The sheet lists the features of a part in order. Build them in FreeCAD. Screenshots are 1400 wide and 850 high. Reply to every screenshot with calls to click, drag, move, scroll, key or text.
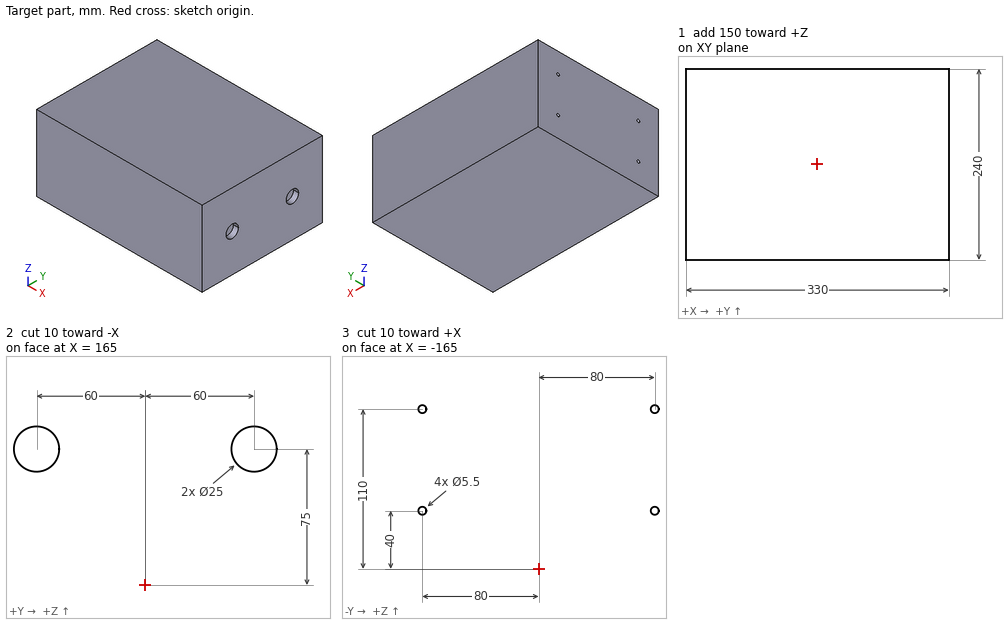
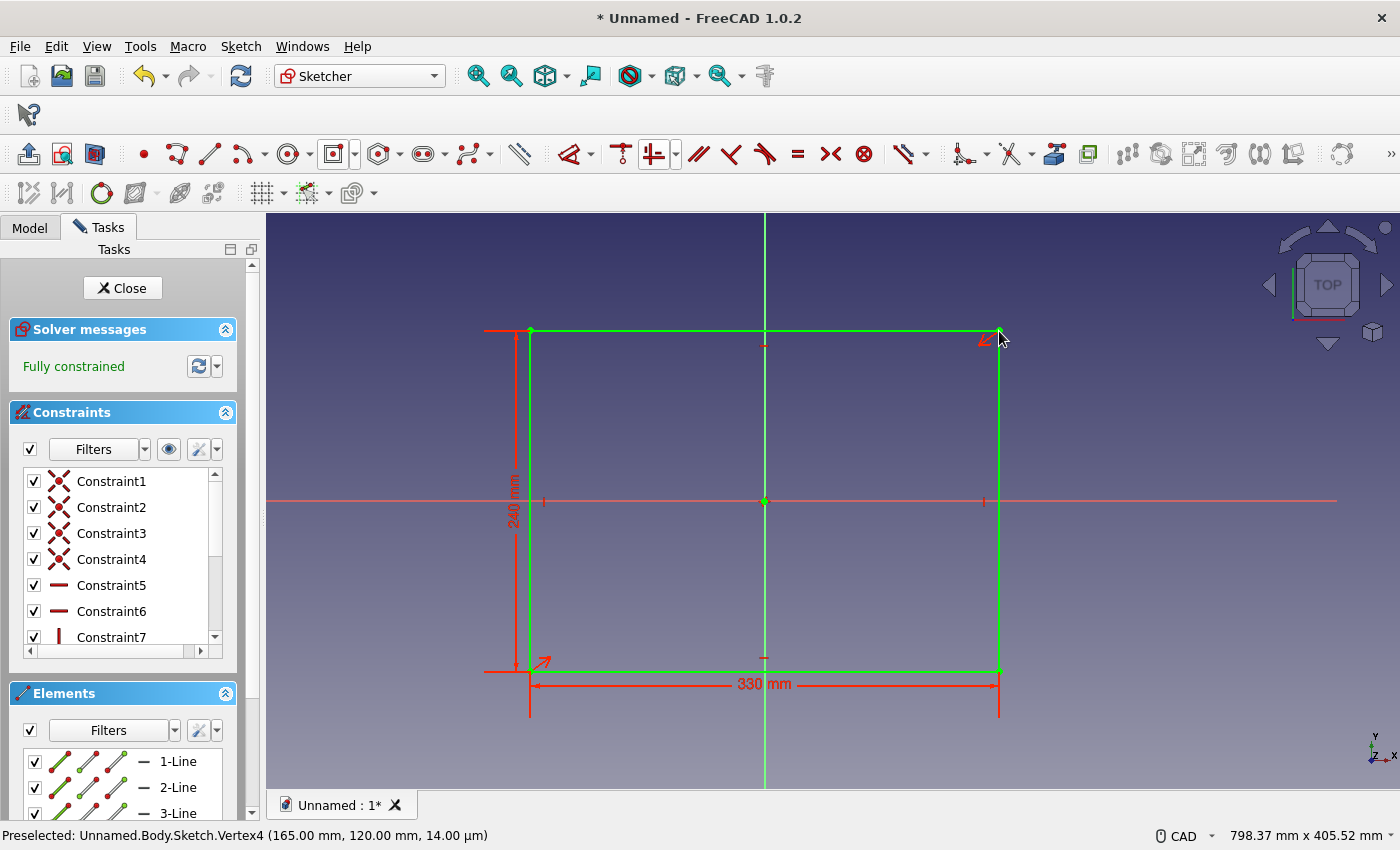
click(123, 288)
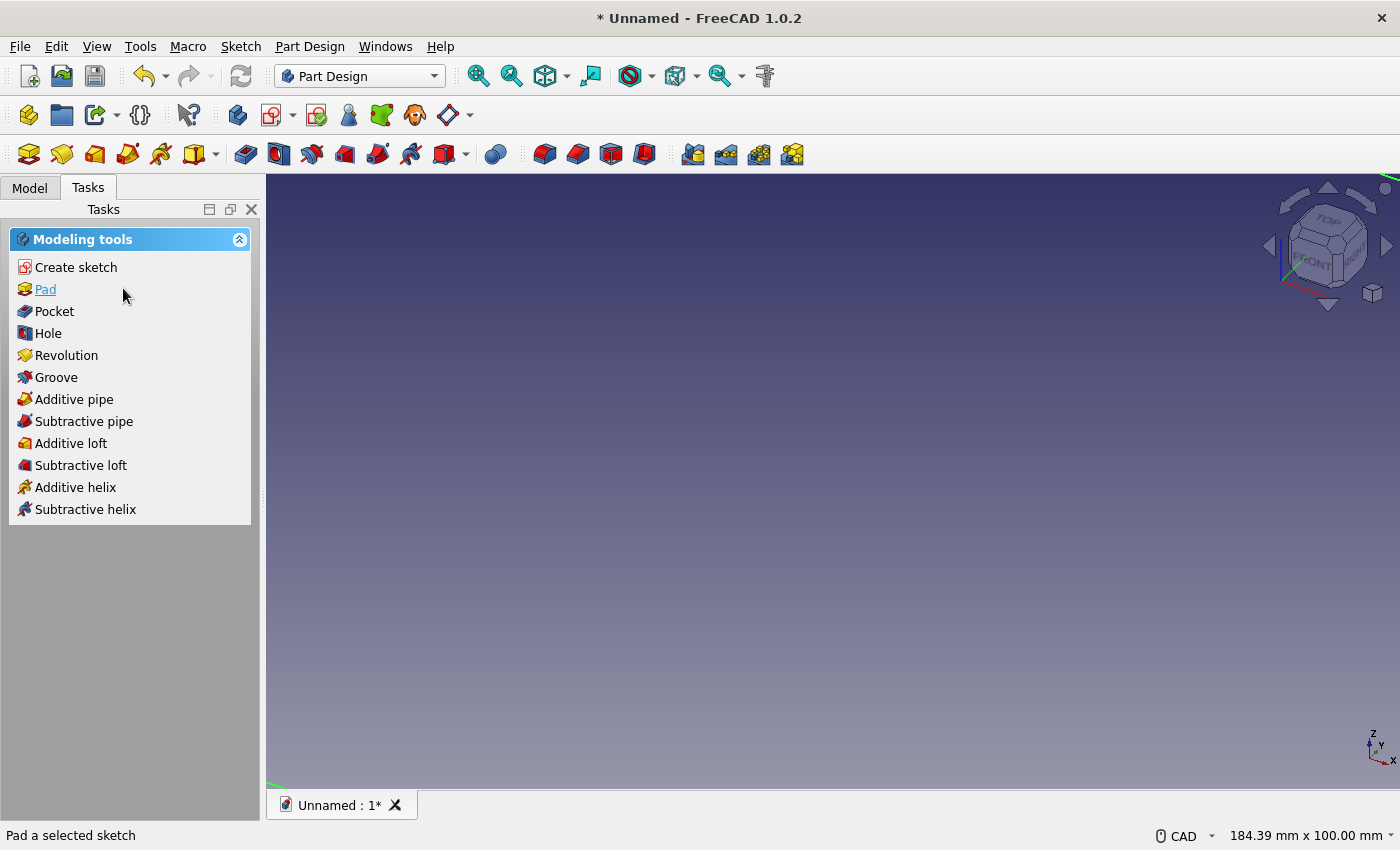
click(29, 154)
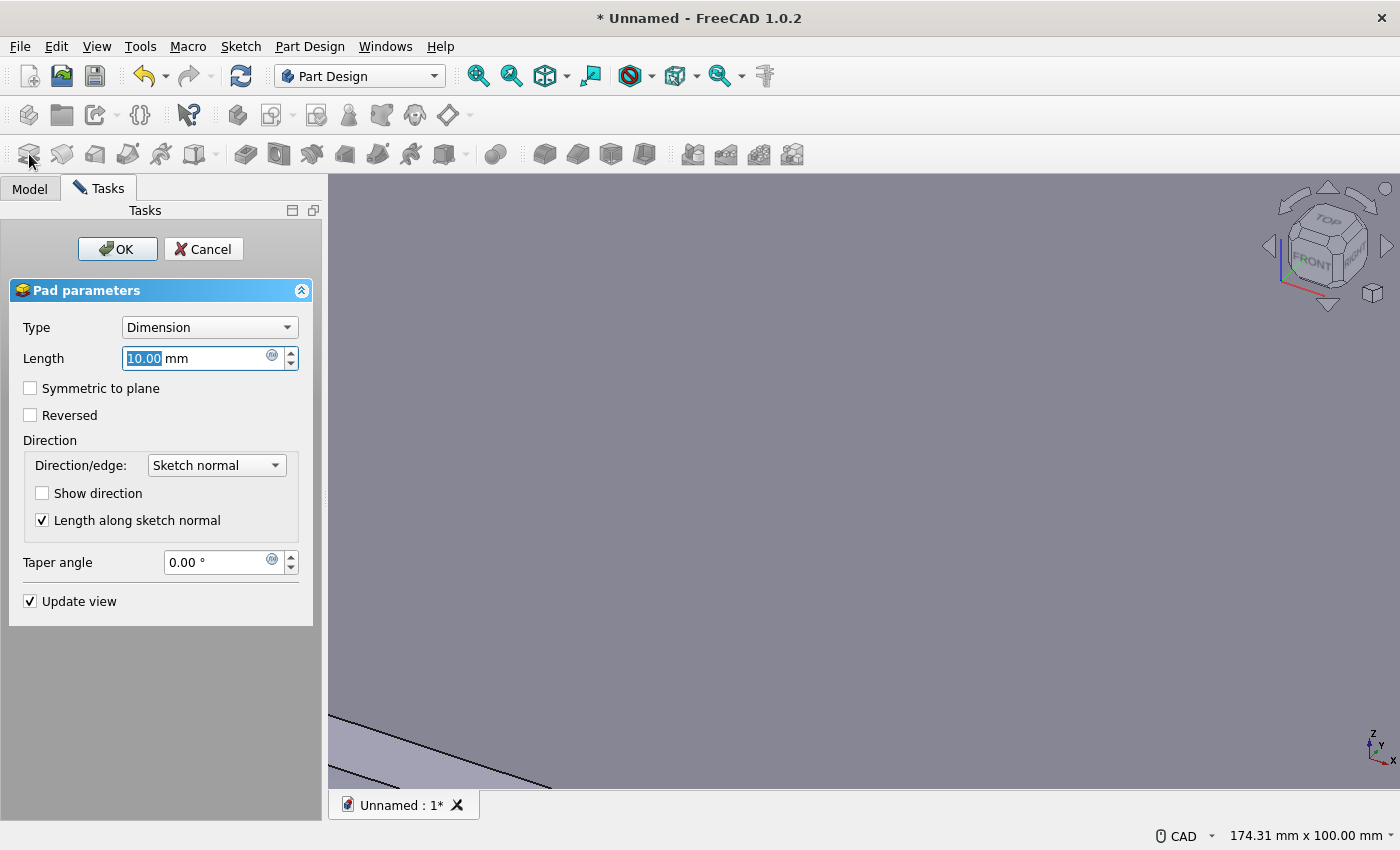
text(150)
key(Tab)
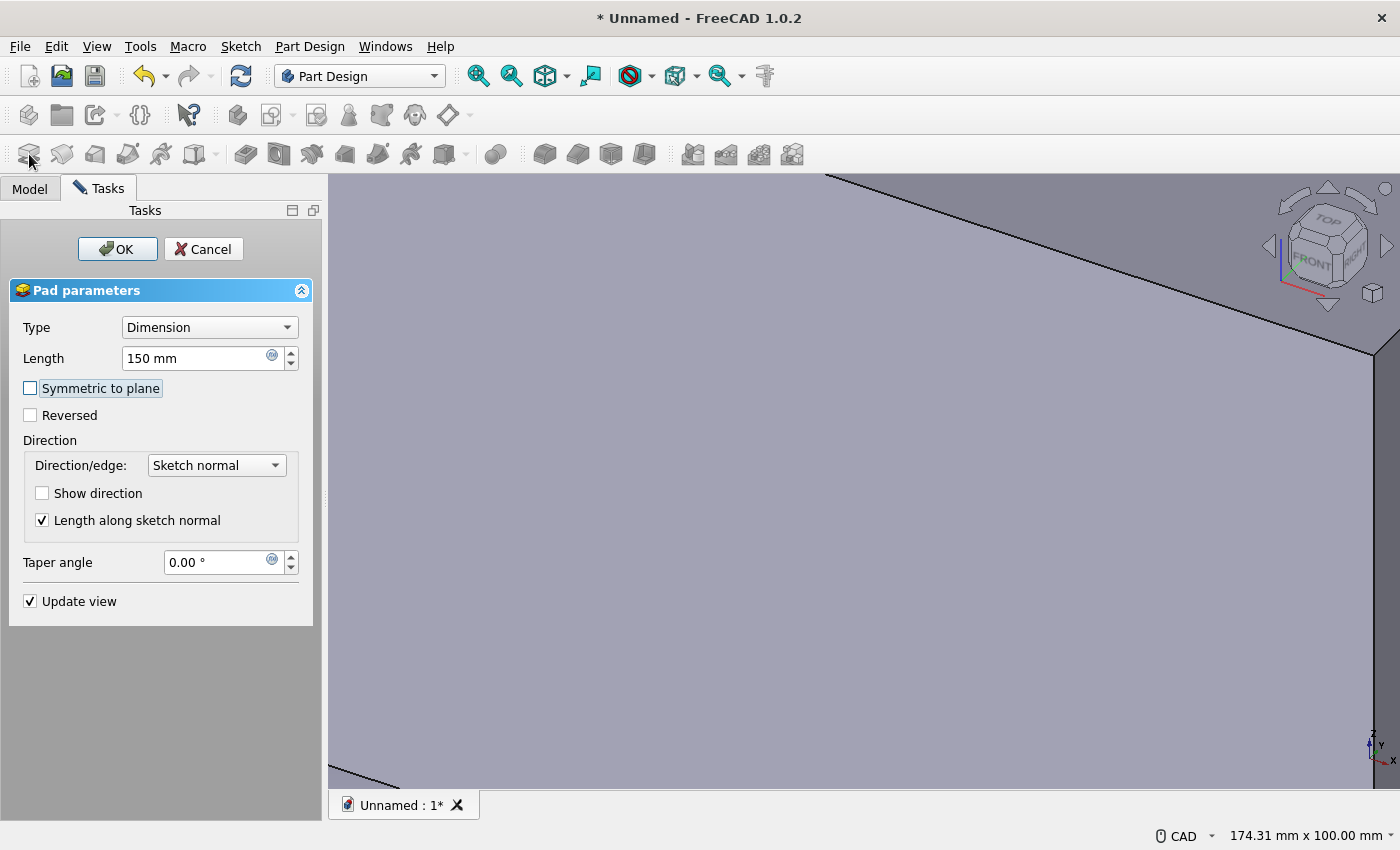
click(118, 249)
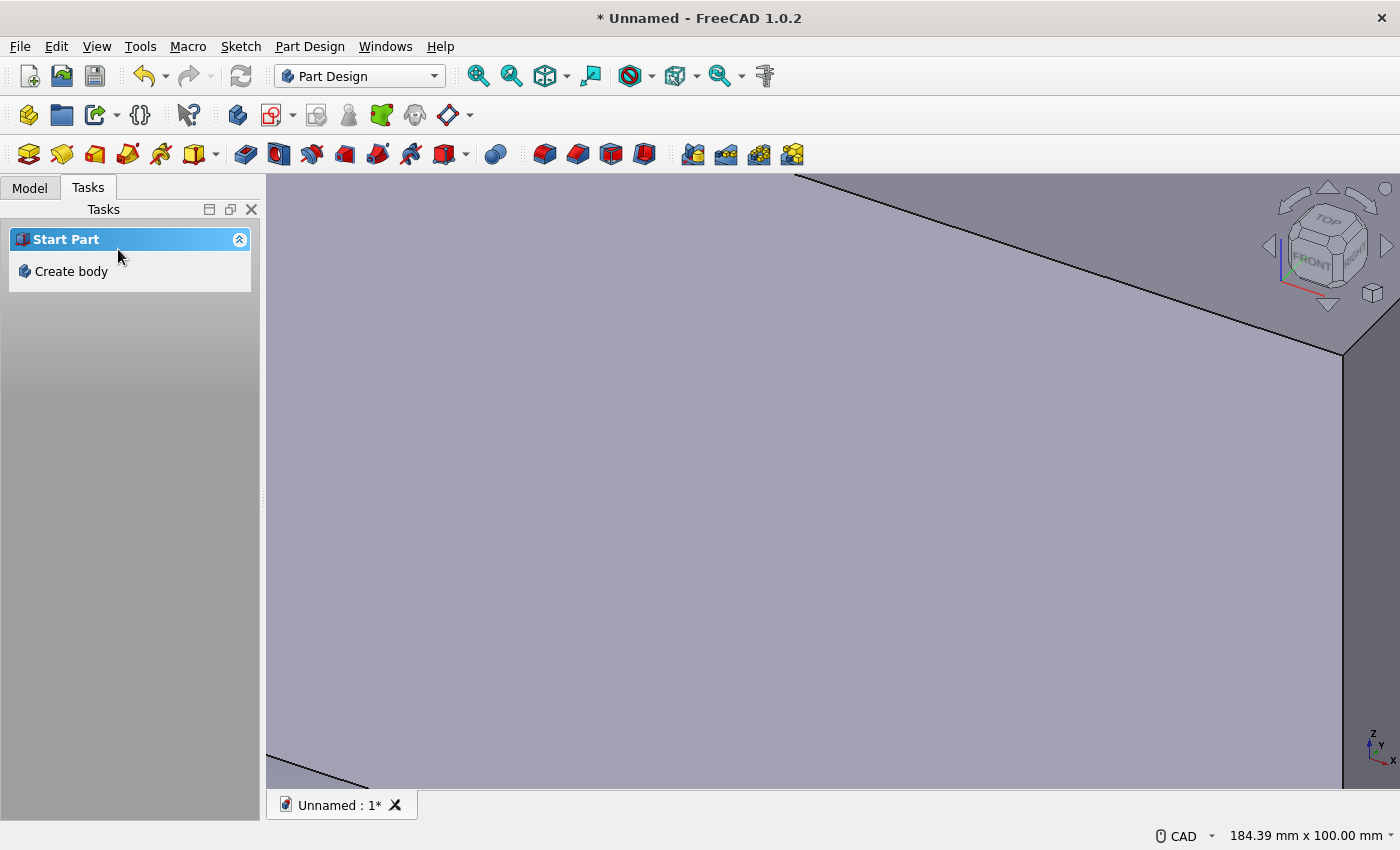
click(479, 76)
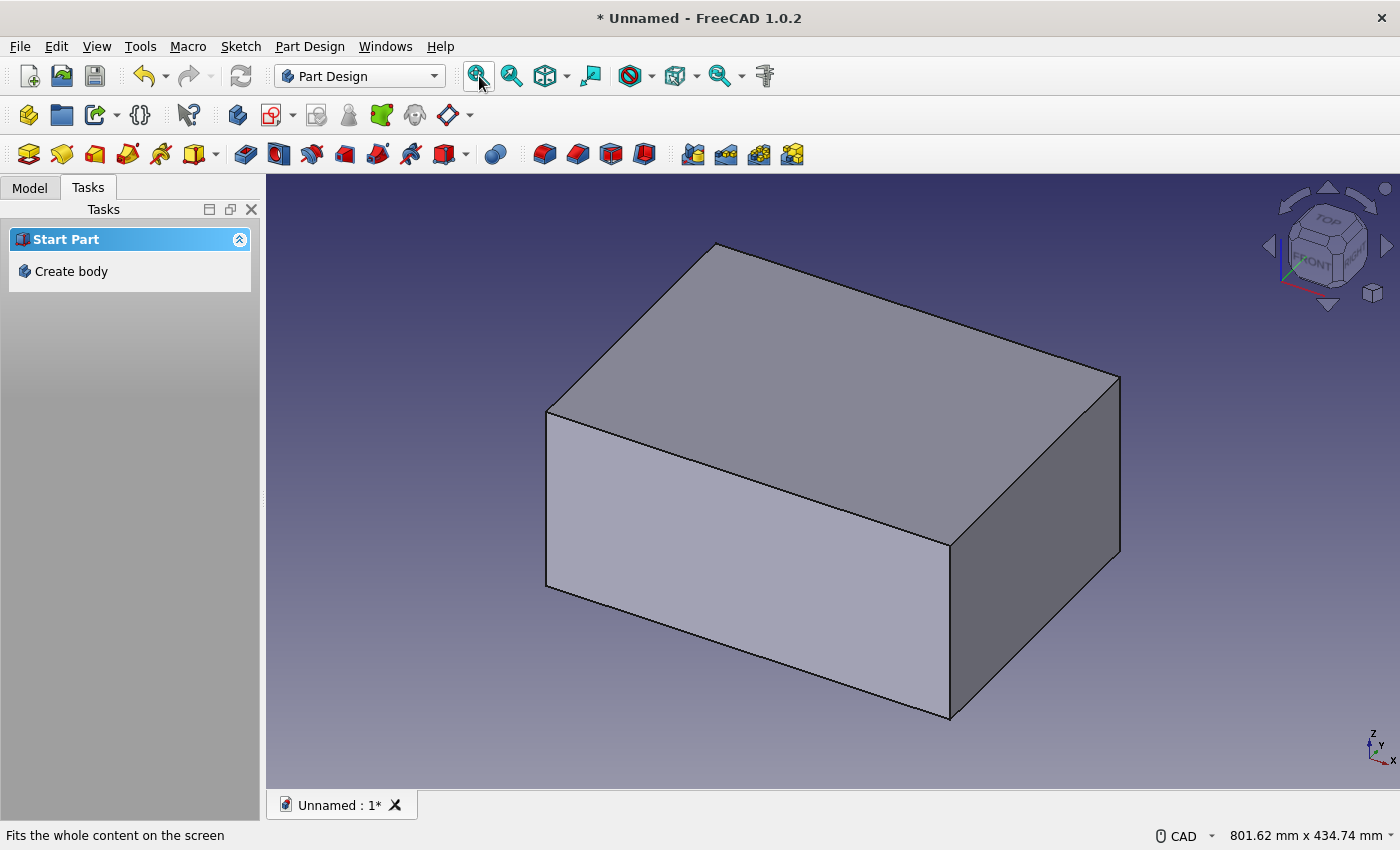
click(1059, 523)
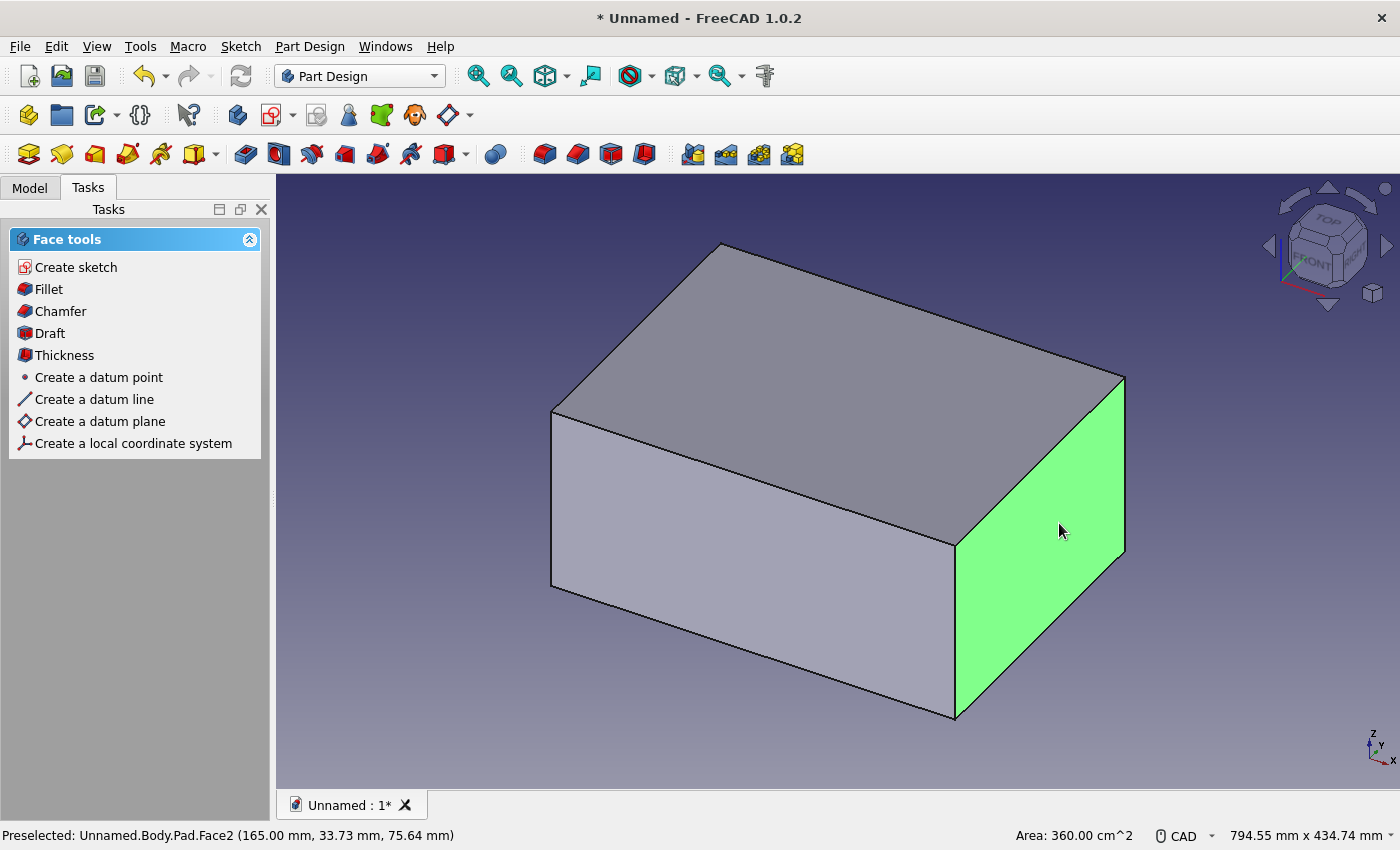
click(270, 116)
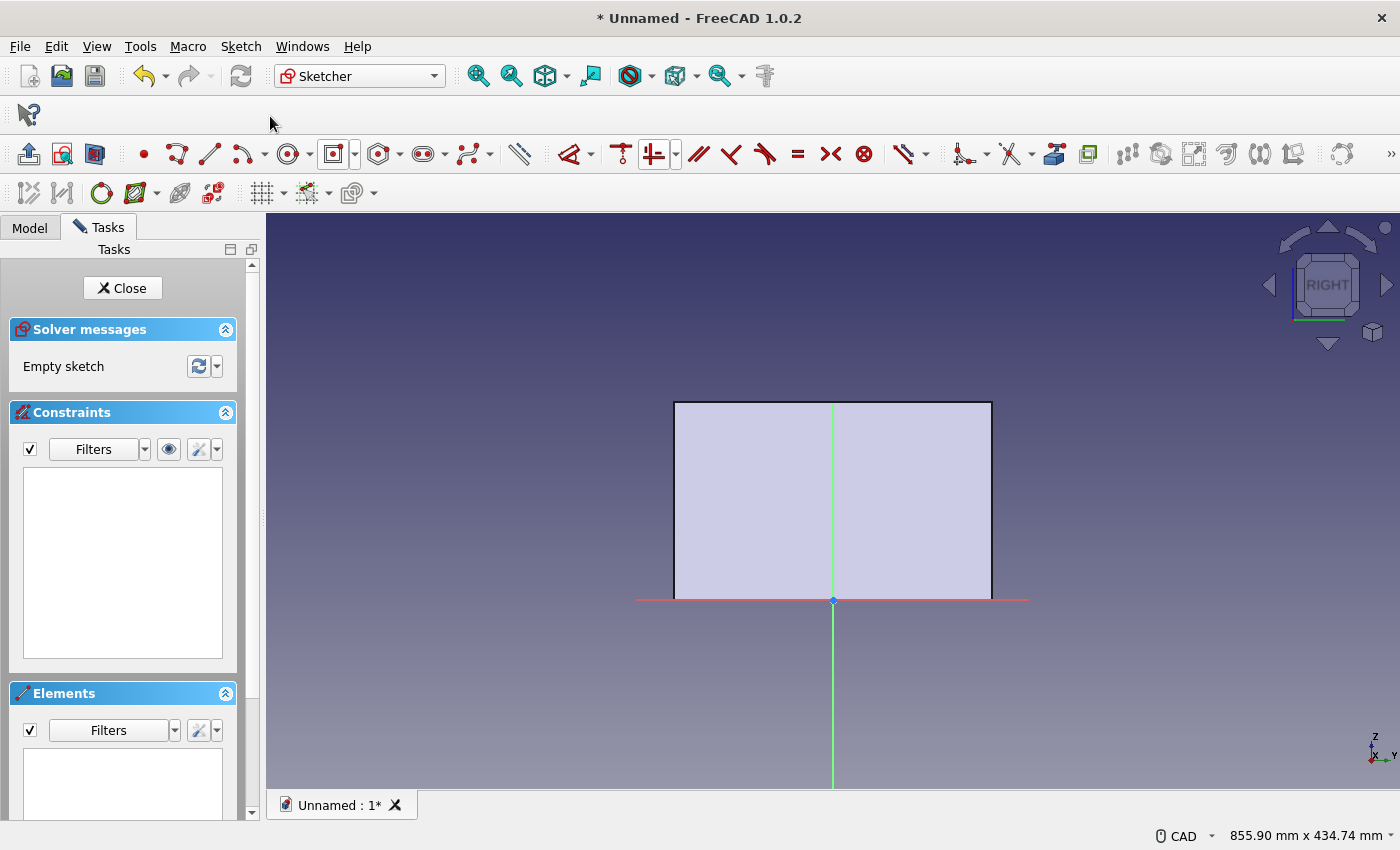
scroll(863, 560, up, 6)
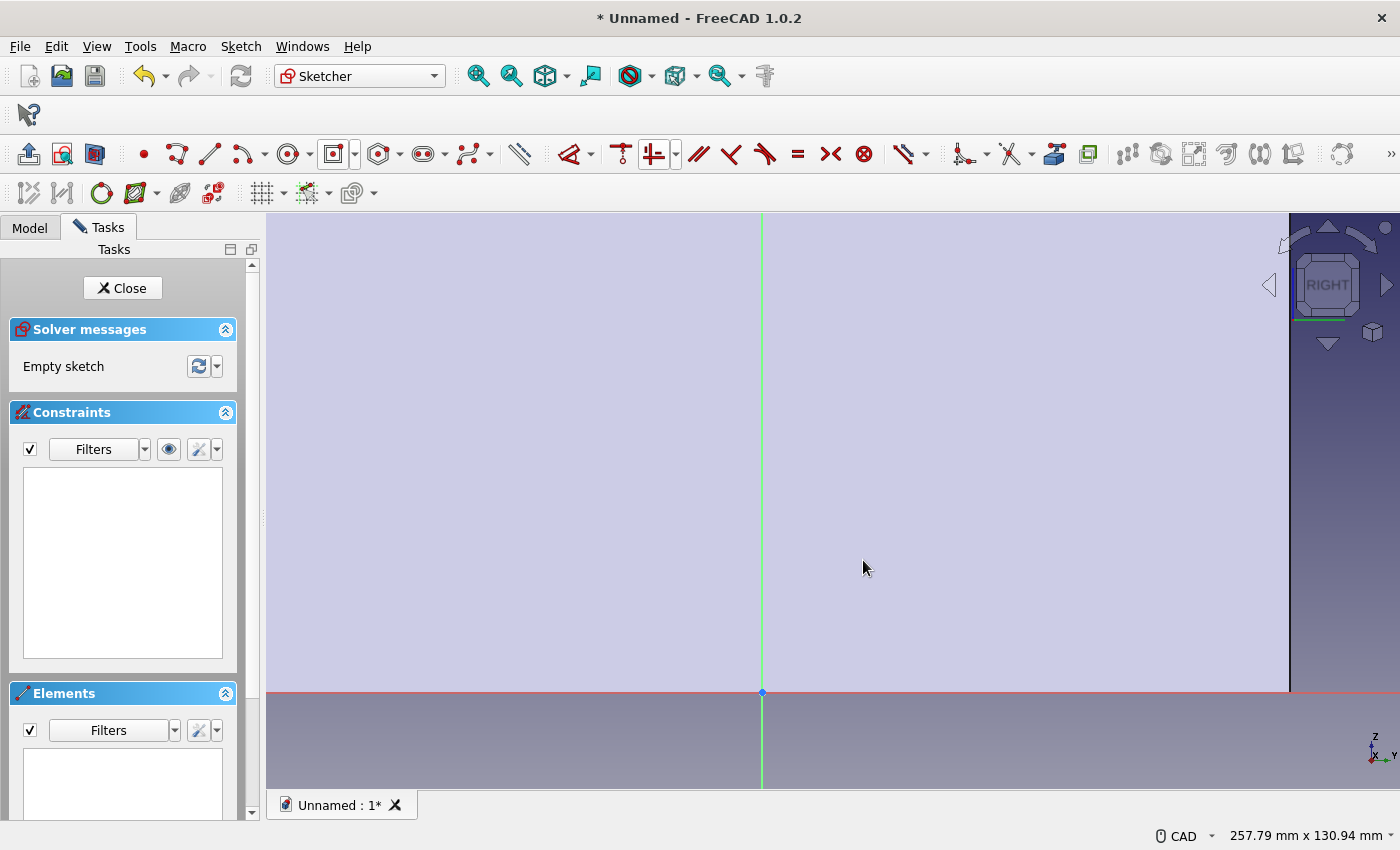
click(288, 154)